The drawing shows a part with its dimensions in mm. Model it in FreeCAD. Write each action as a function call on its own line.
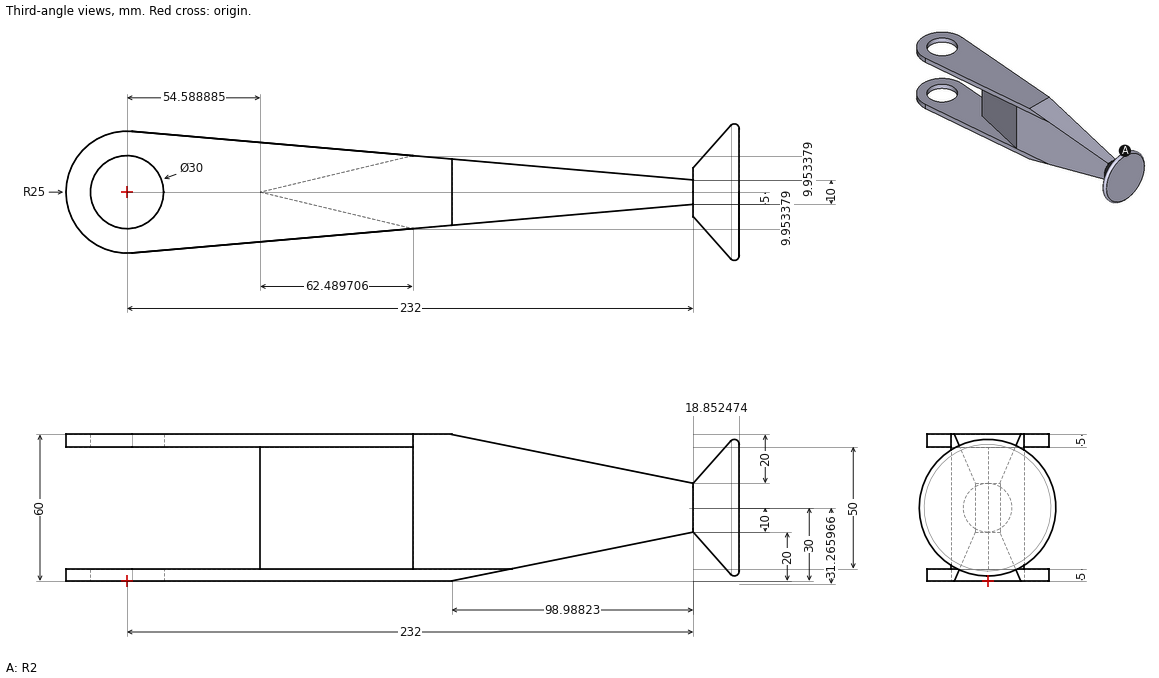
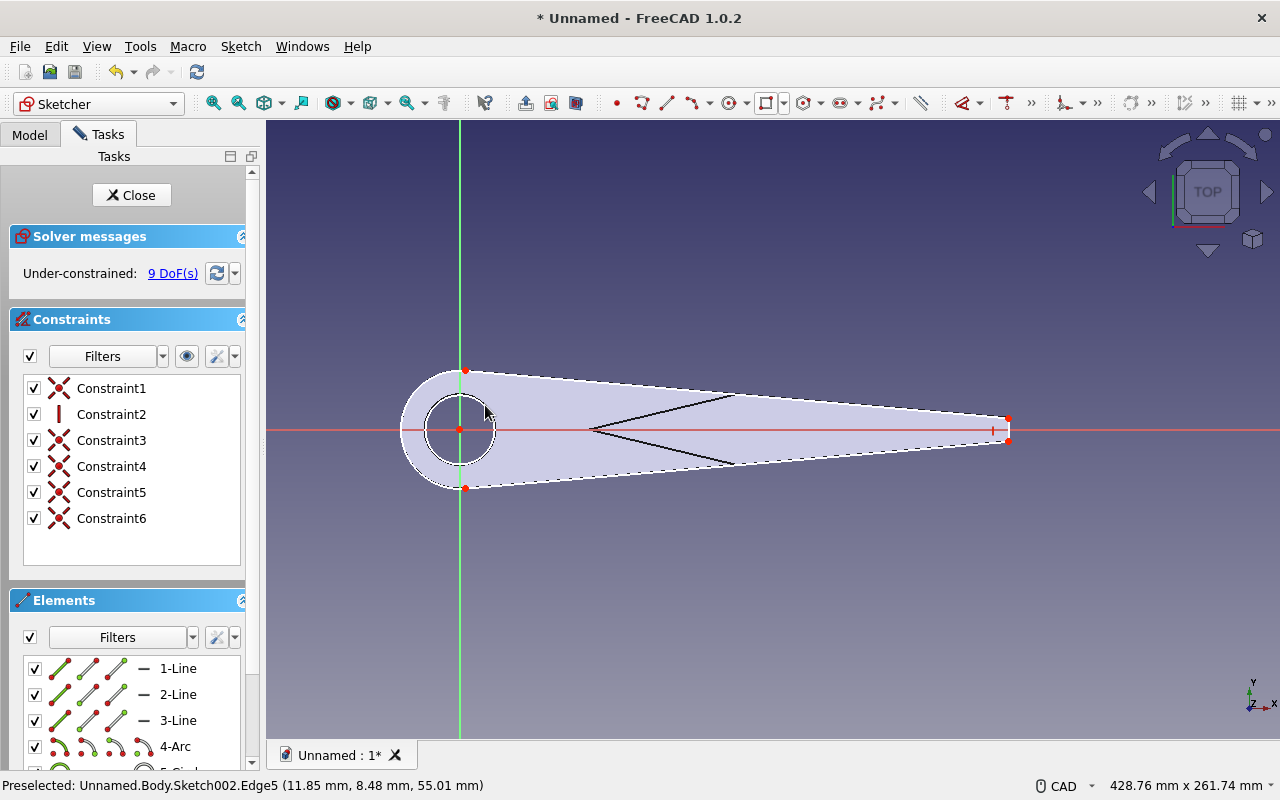
click(628, 475)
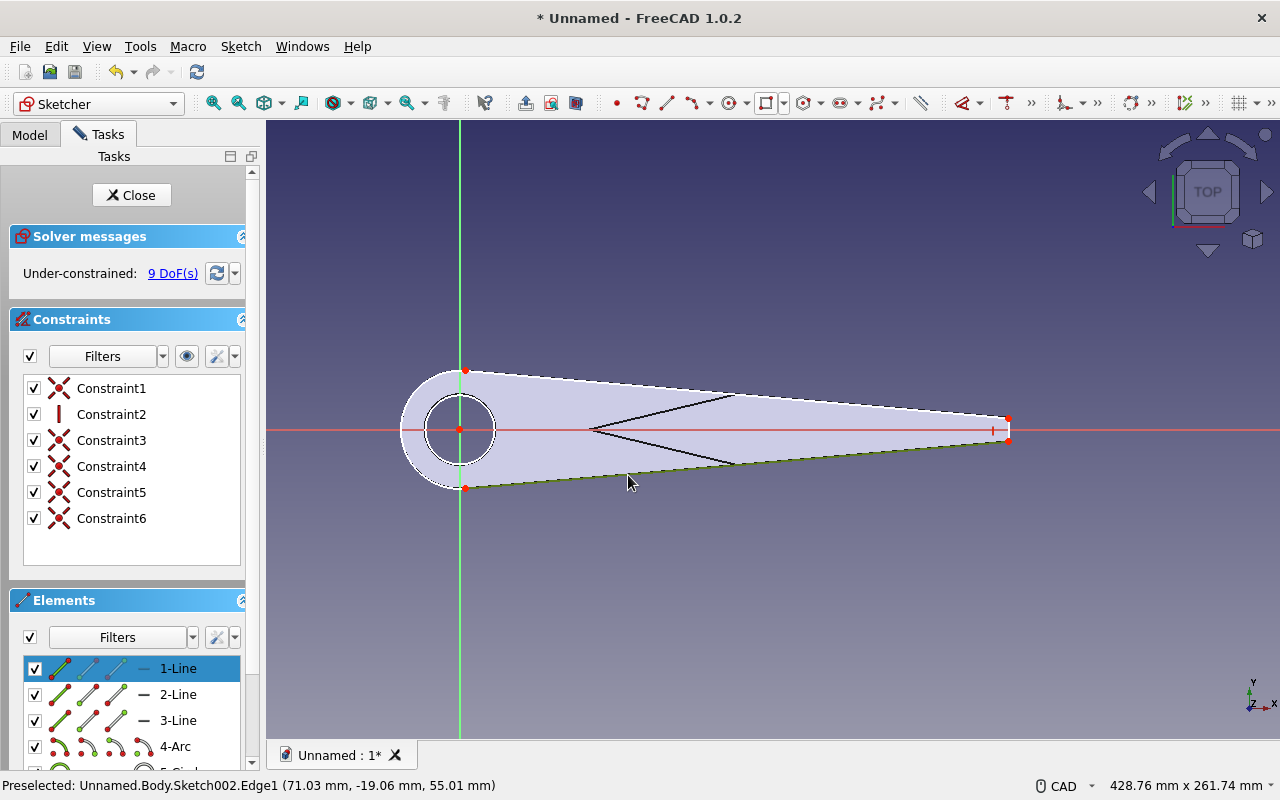
click(413, 393)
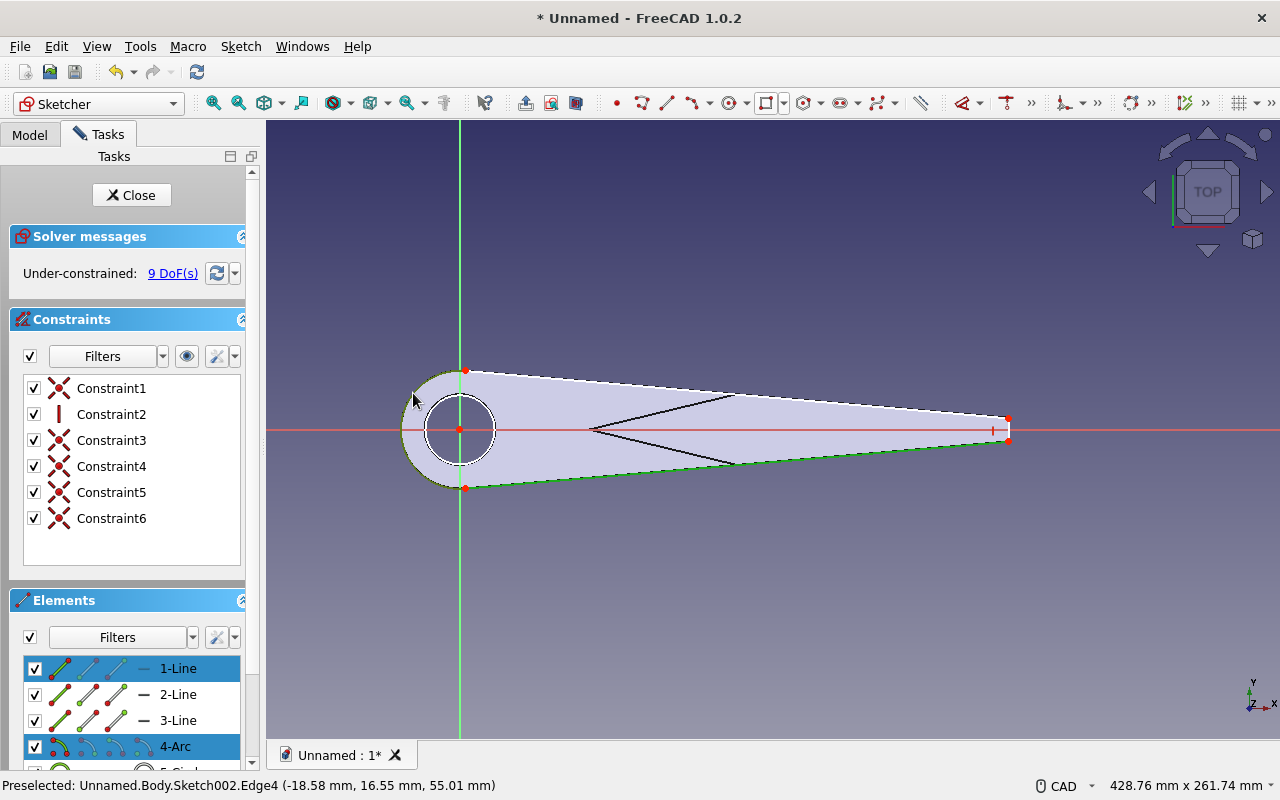
key(t)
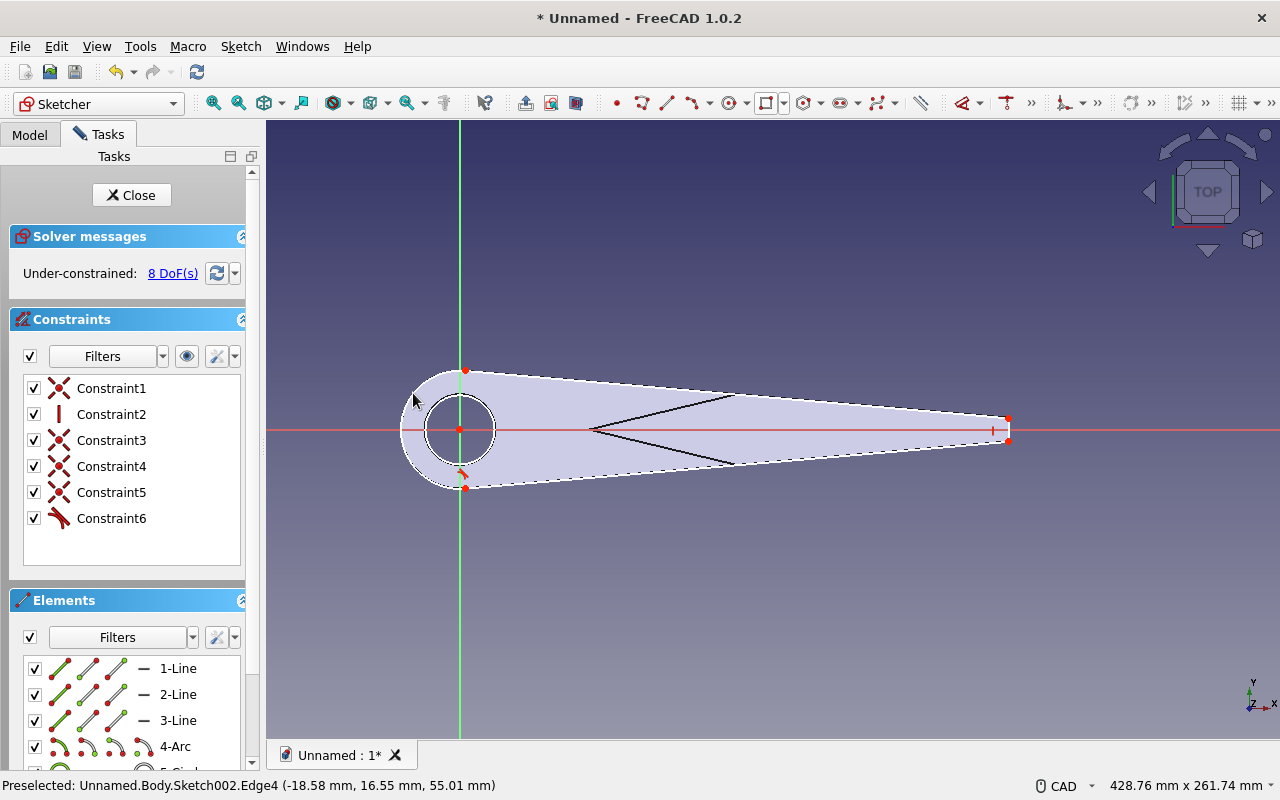
click(846, 404)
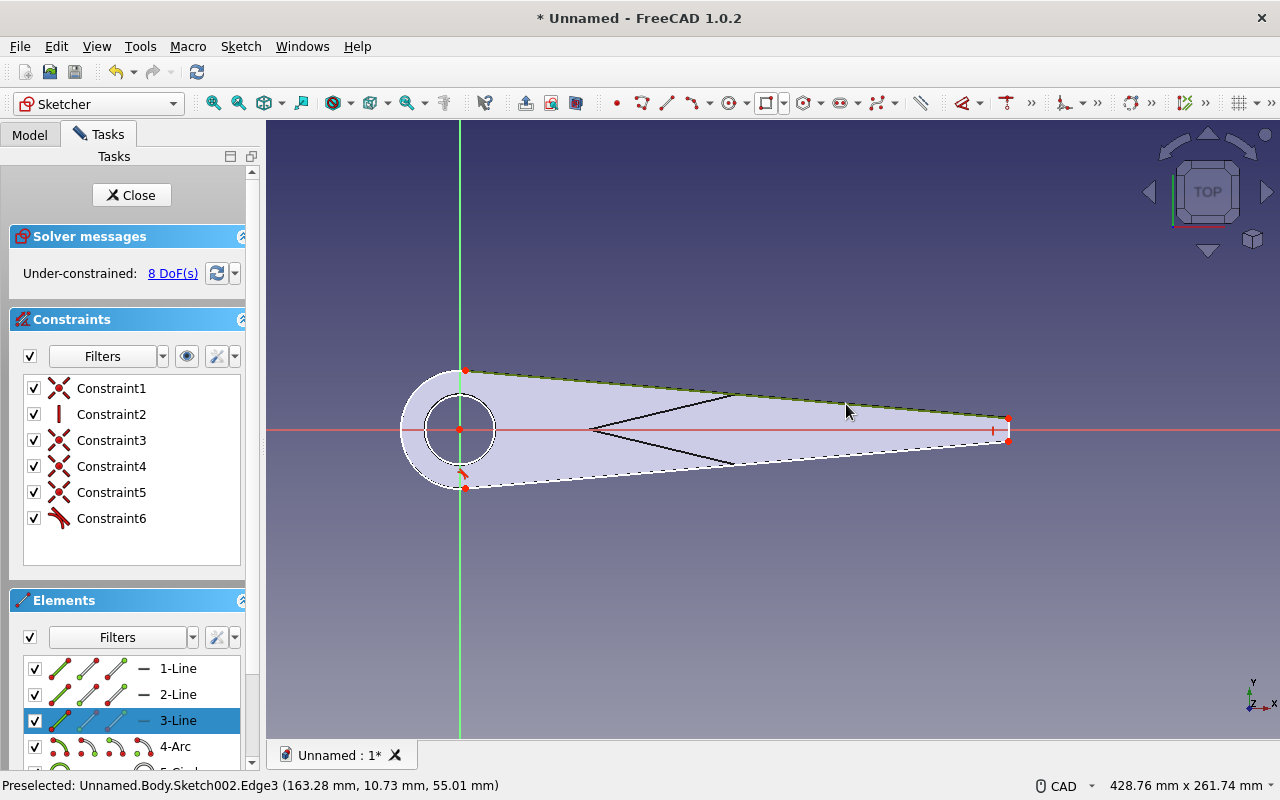
click(413, 393)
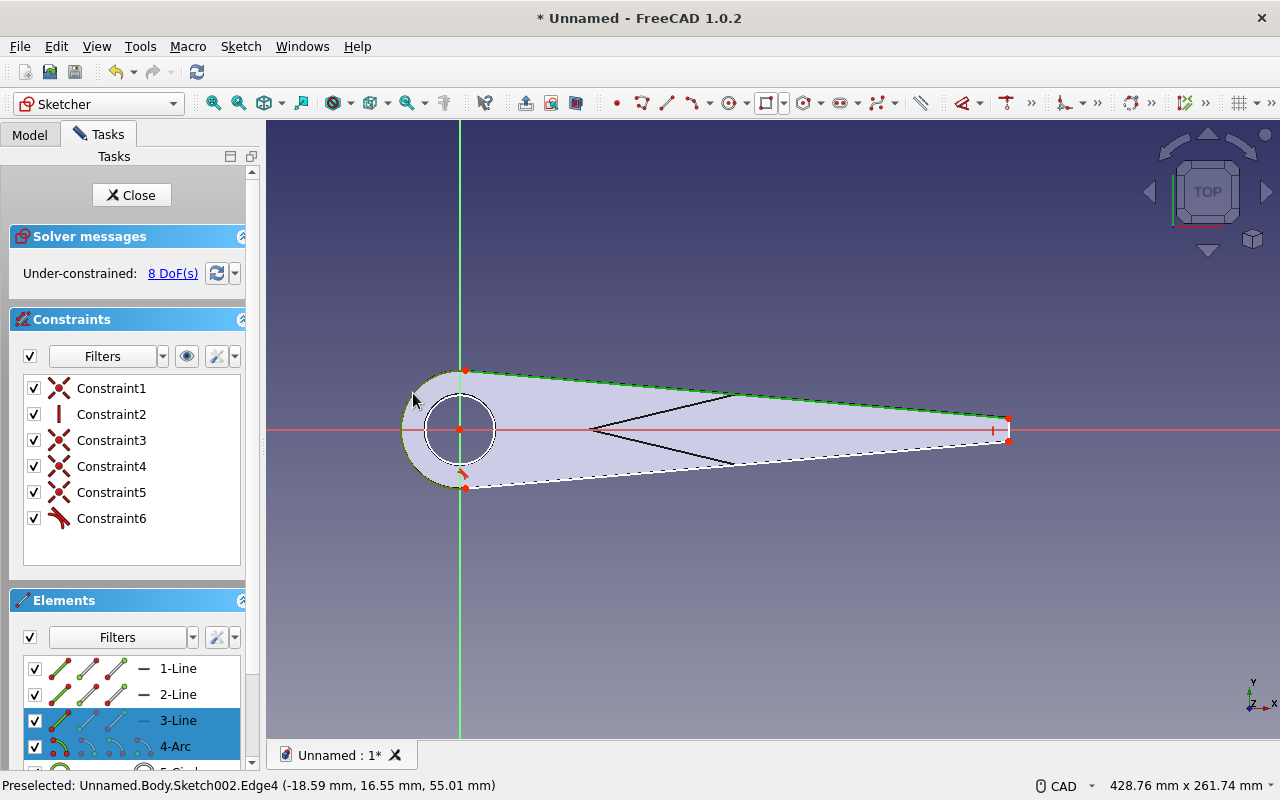
key(t)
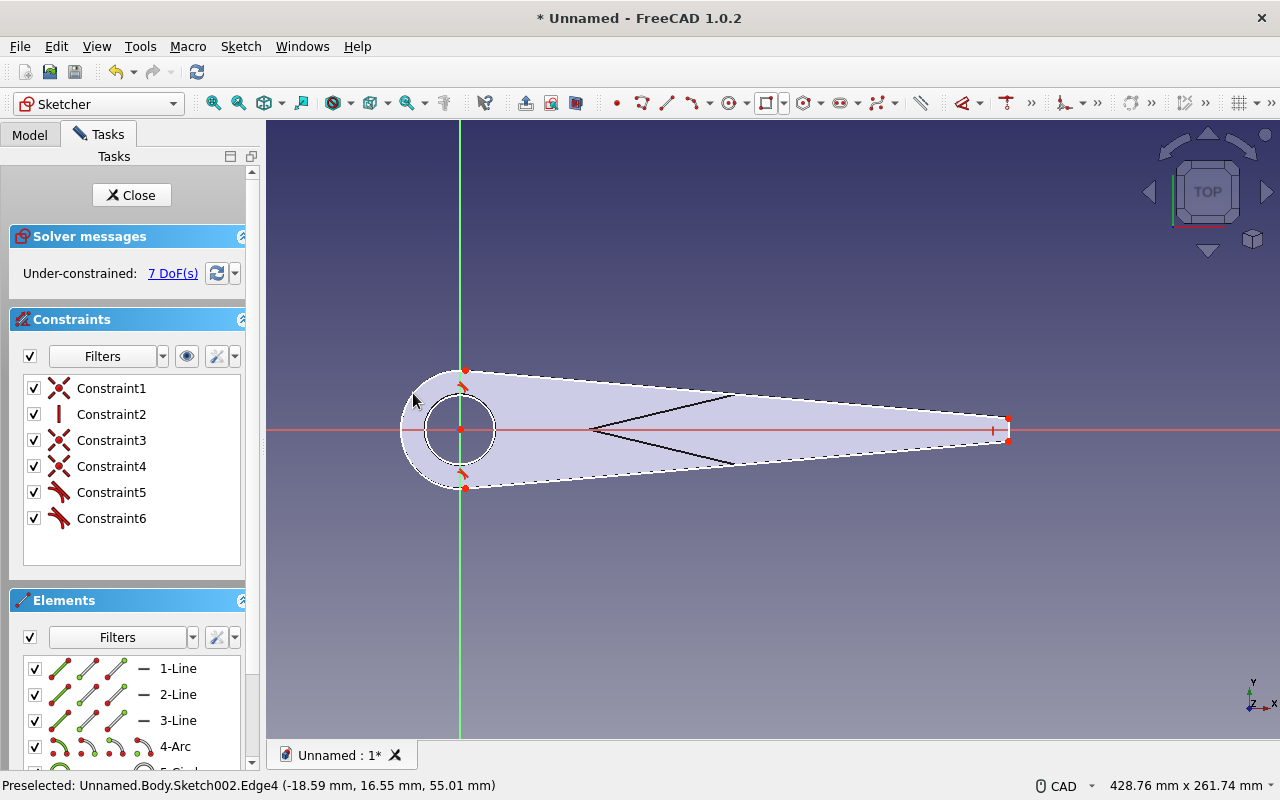
drag(450, 420, 470, 440)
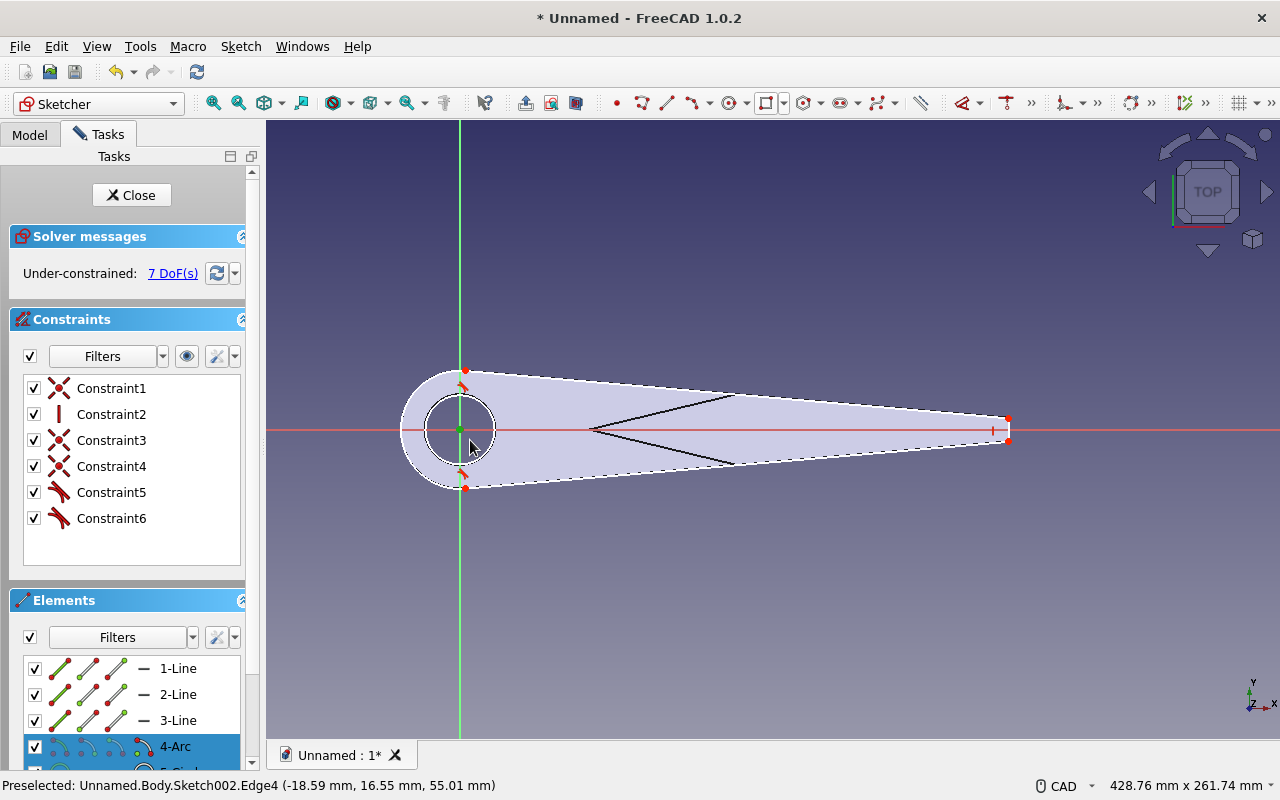
click(1006, 104)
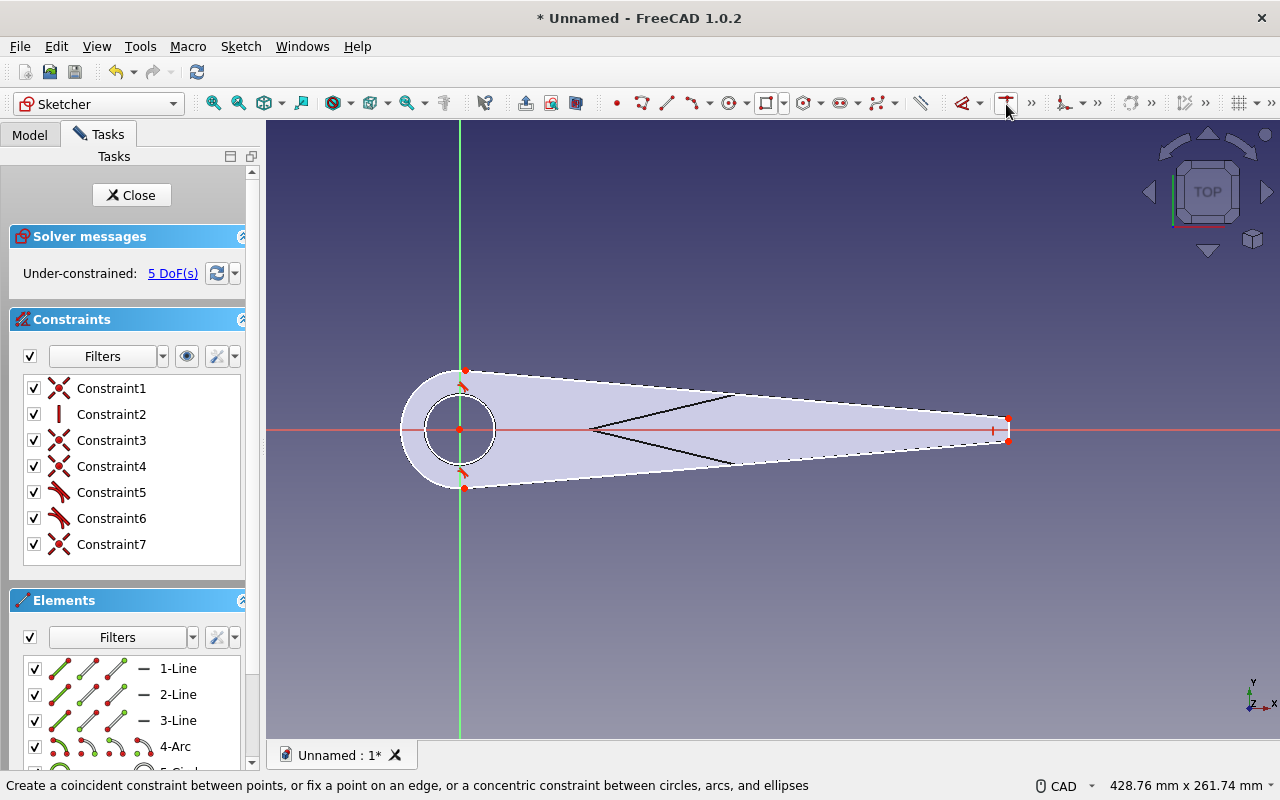
click(962, 104)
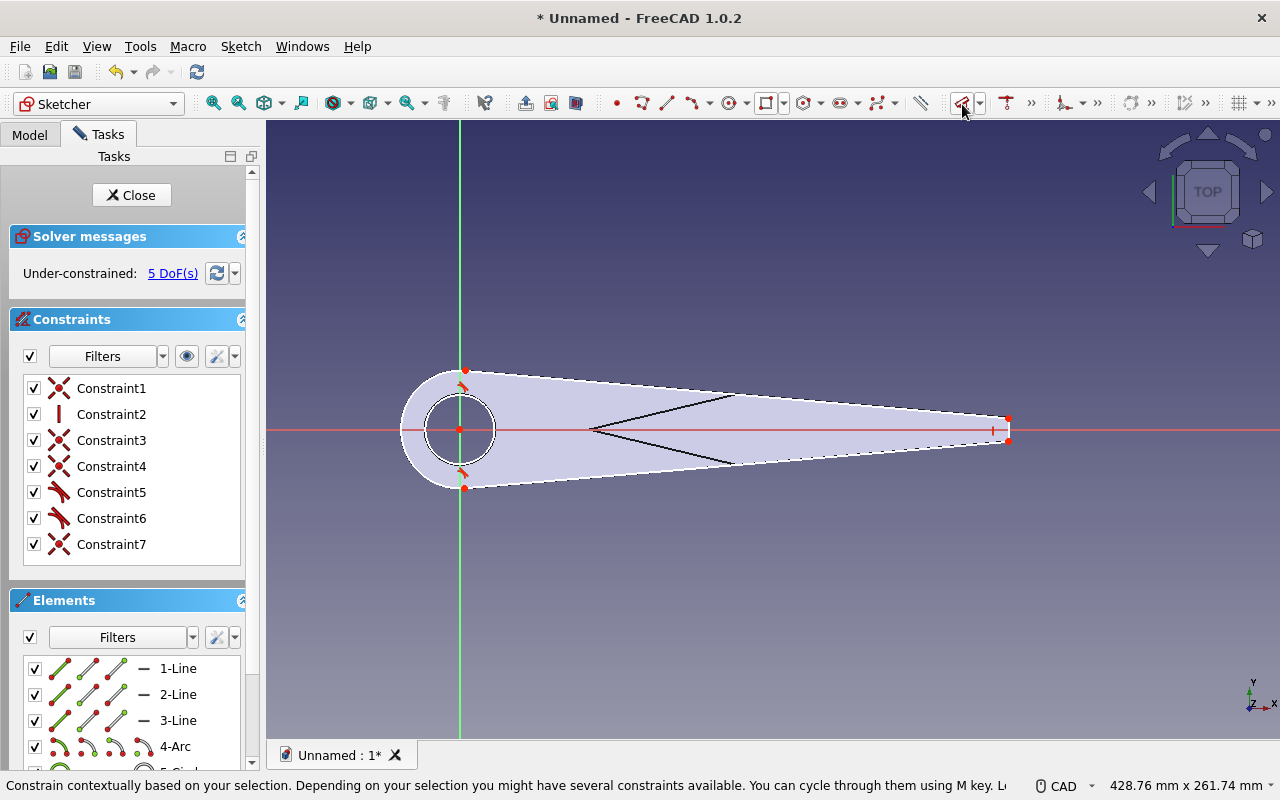
click(414, 393)
click(389, 373)